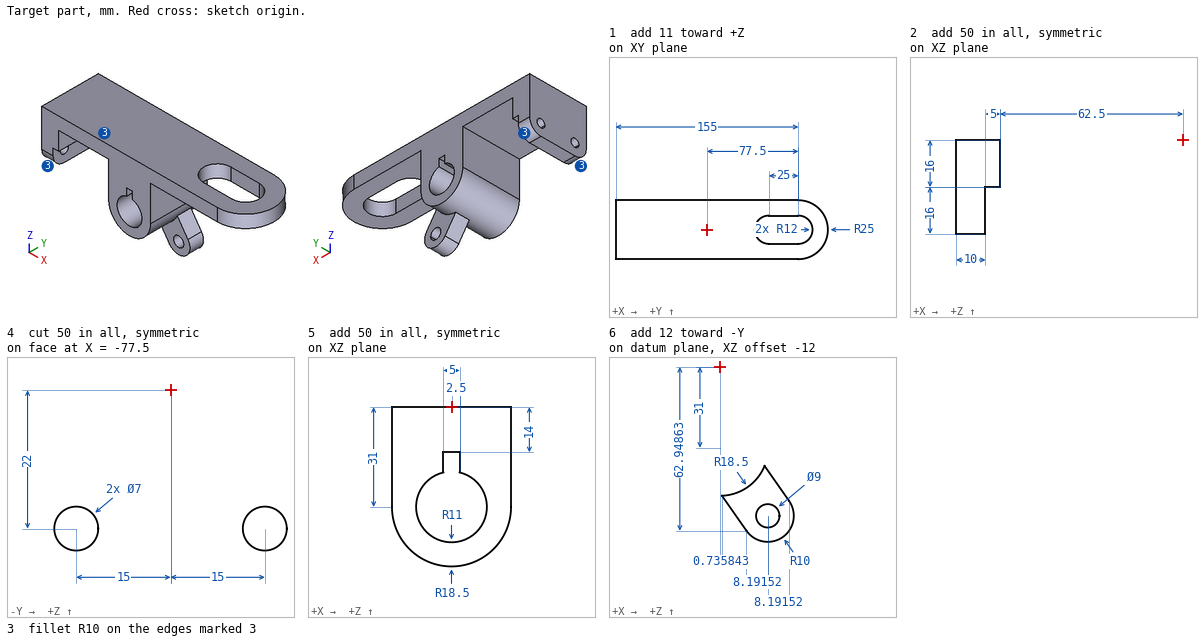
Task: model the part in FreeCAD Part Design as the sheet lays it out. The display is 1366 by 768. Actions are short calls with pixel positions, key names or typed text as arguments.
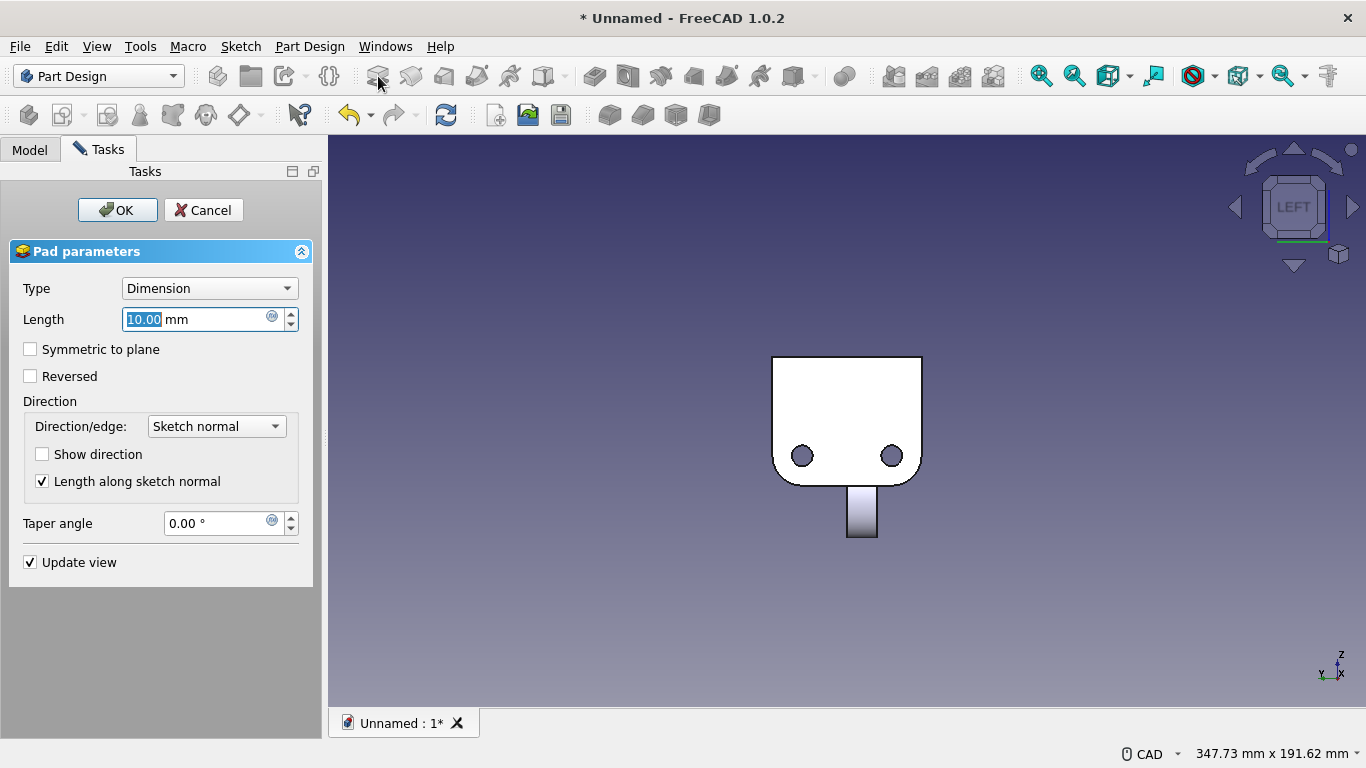
text(50)
key(Tab)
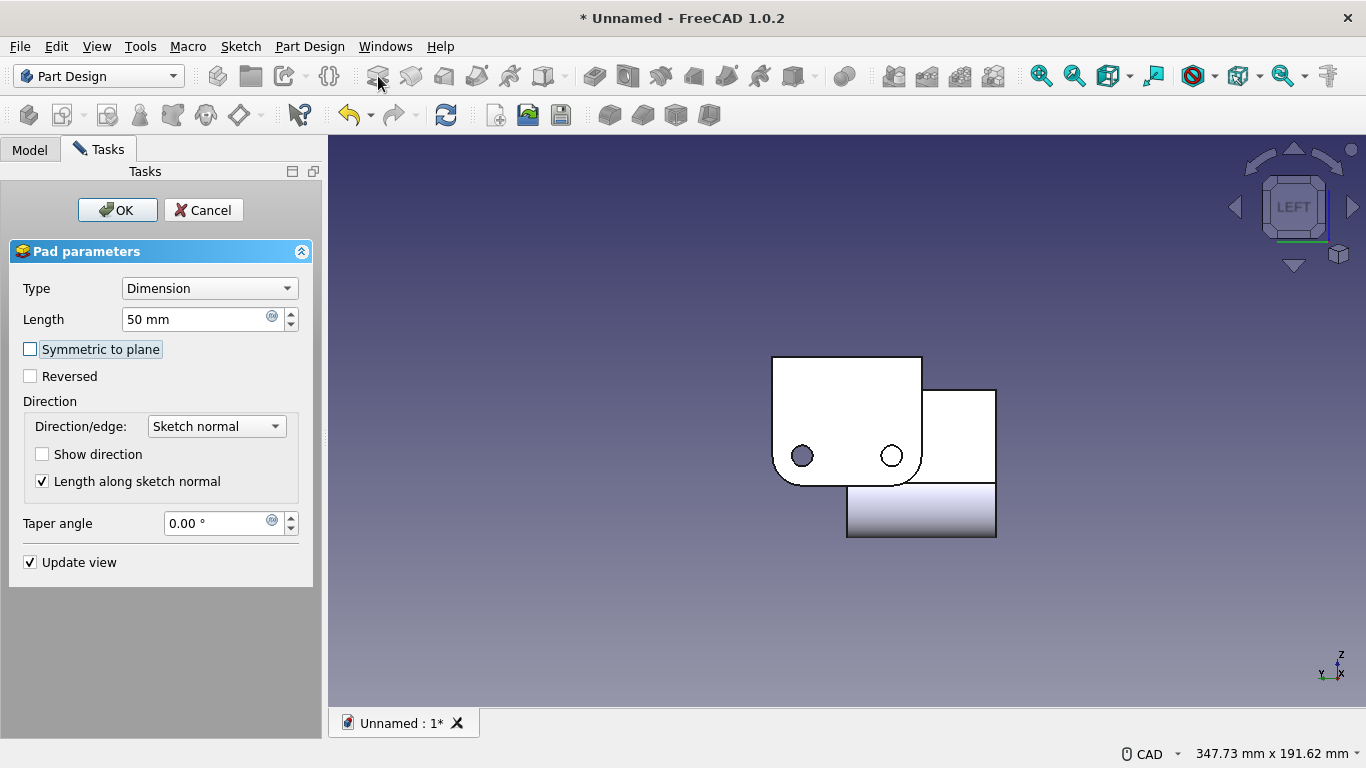
click(31, 349)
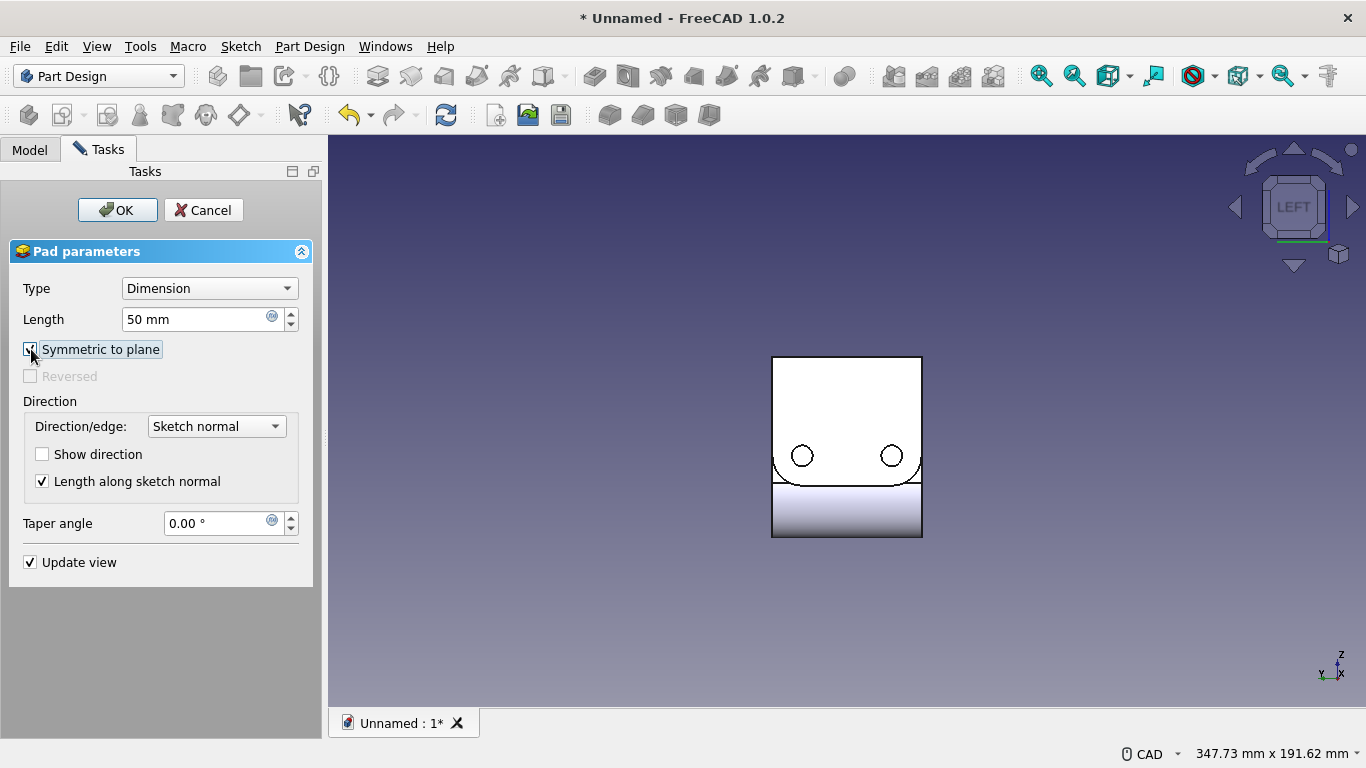
click(118, 210)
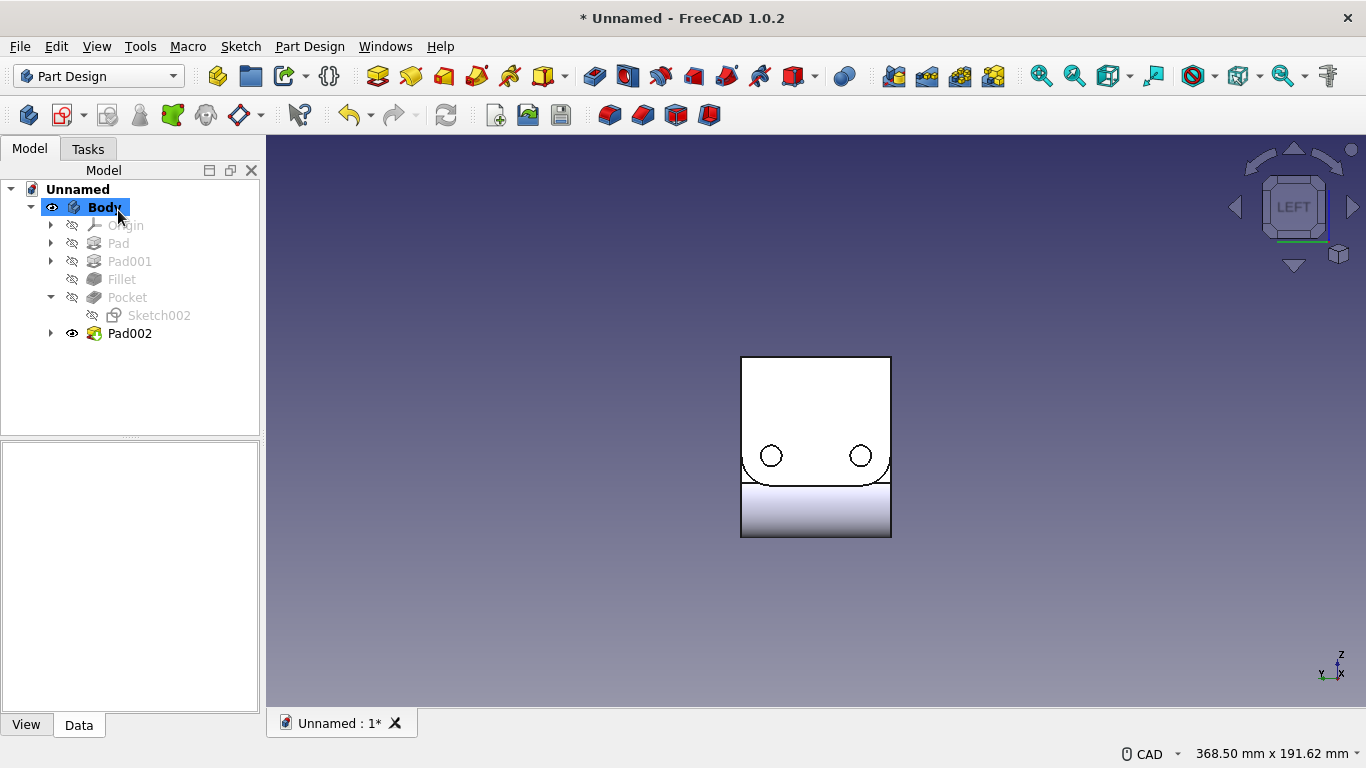
click(1042, 76)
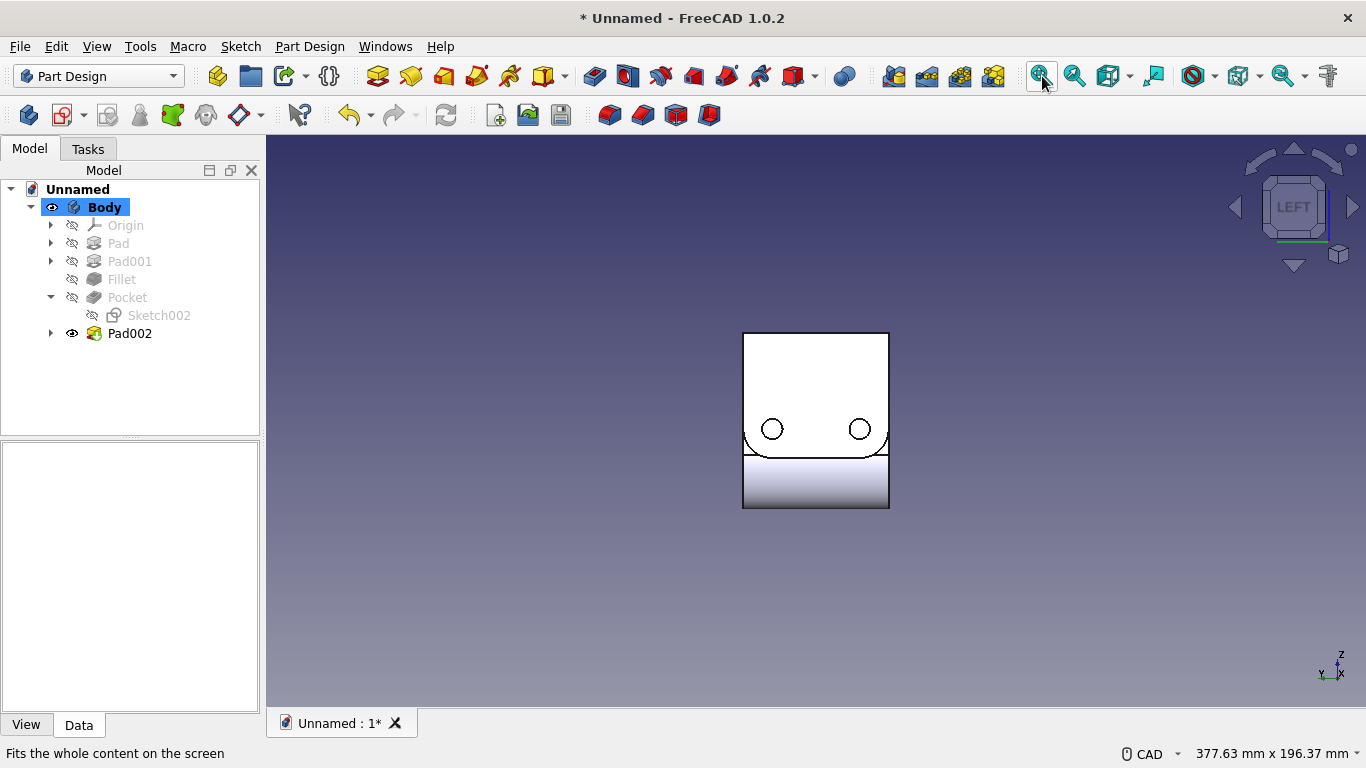
click(51, 225)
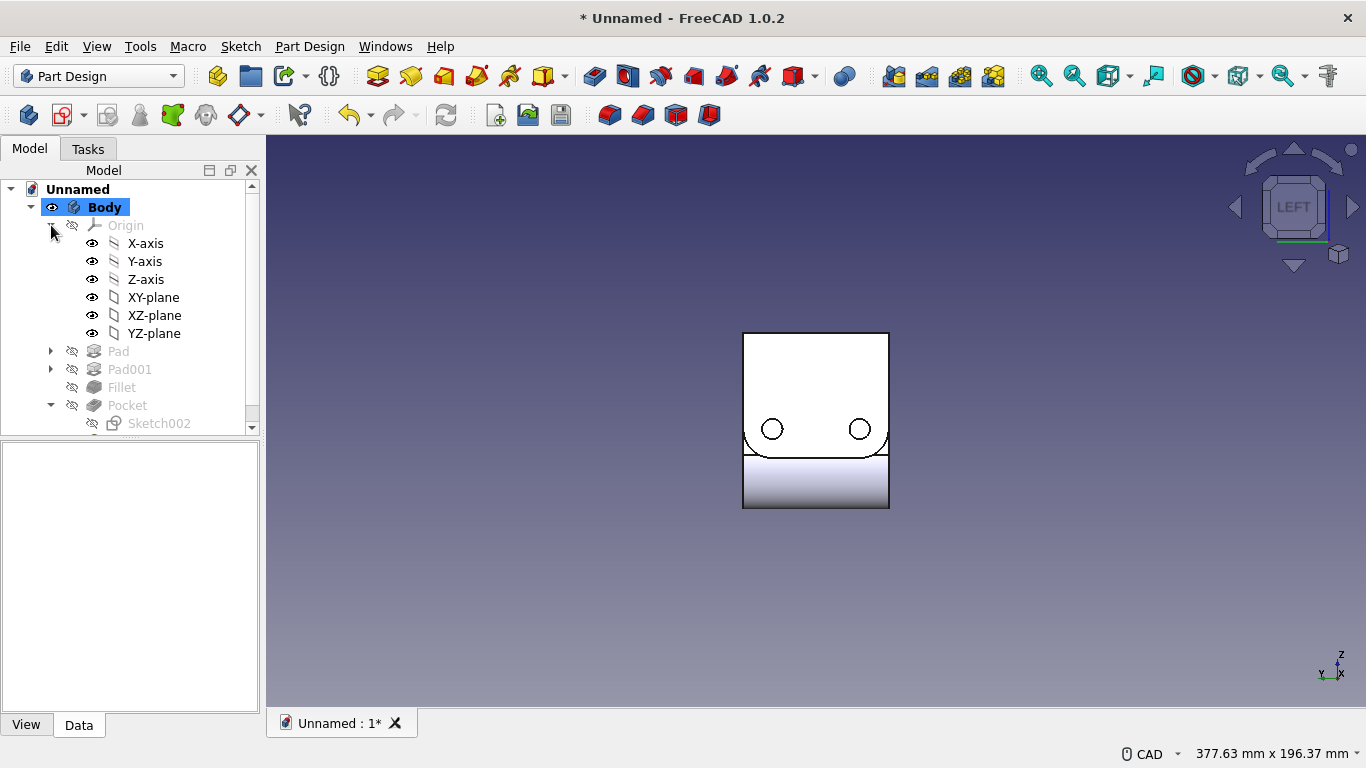
click(137, 315)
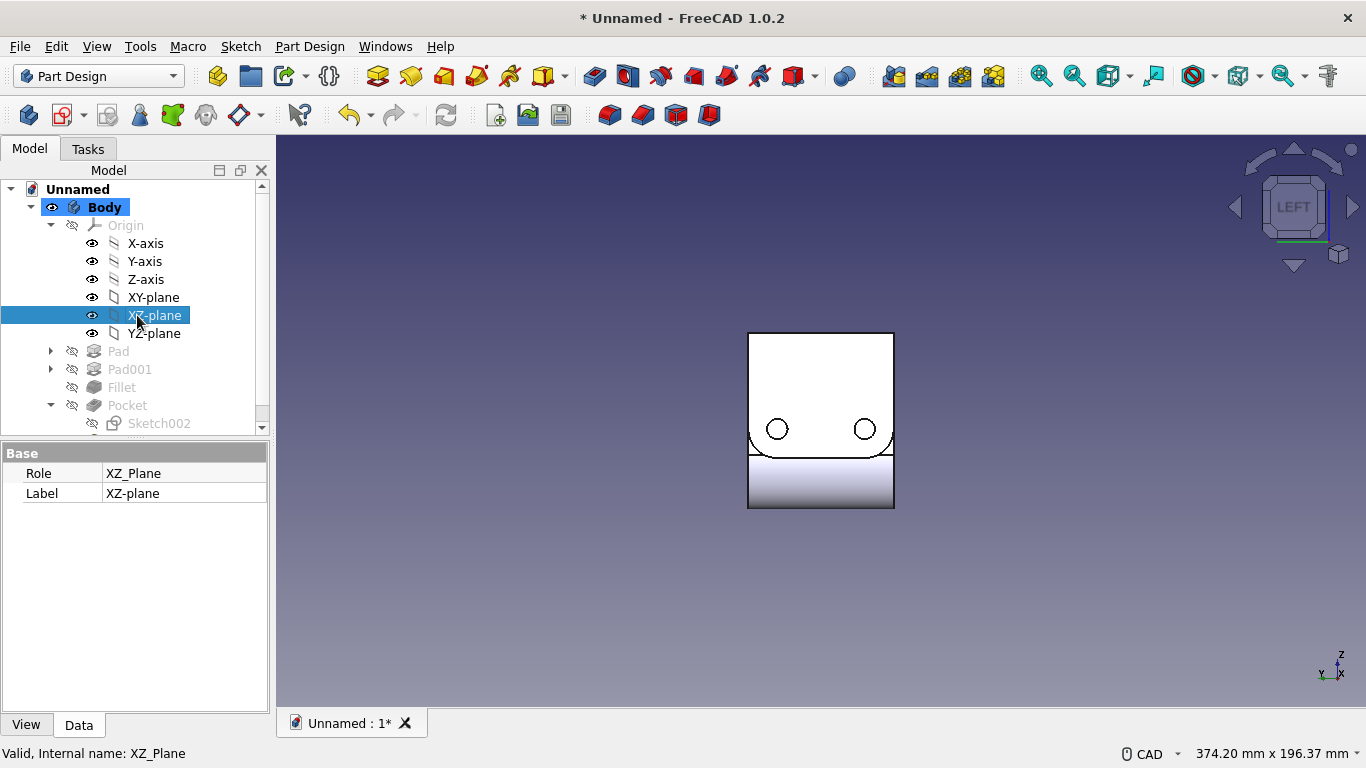
click(238, 116)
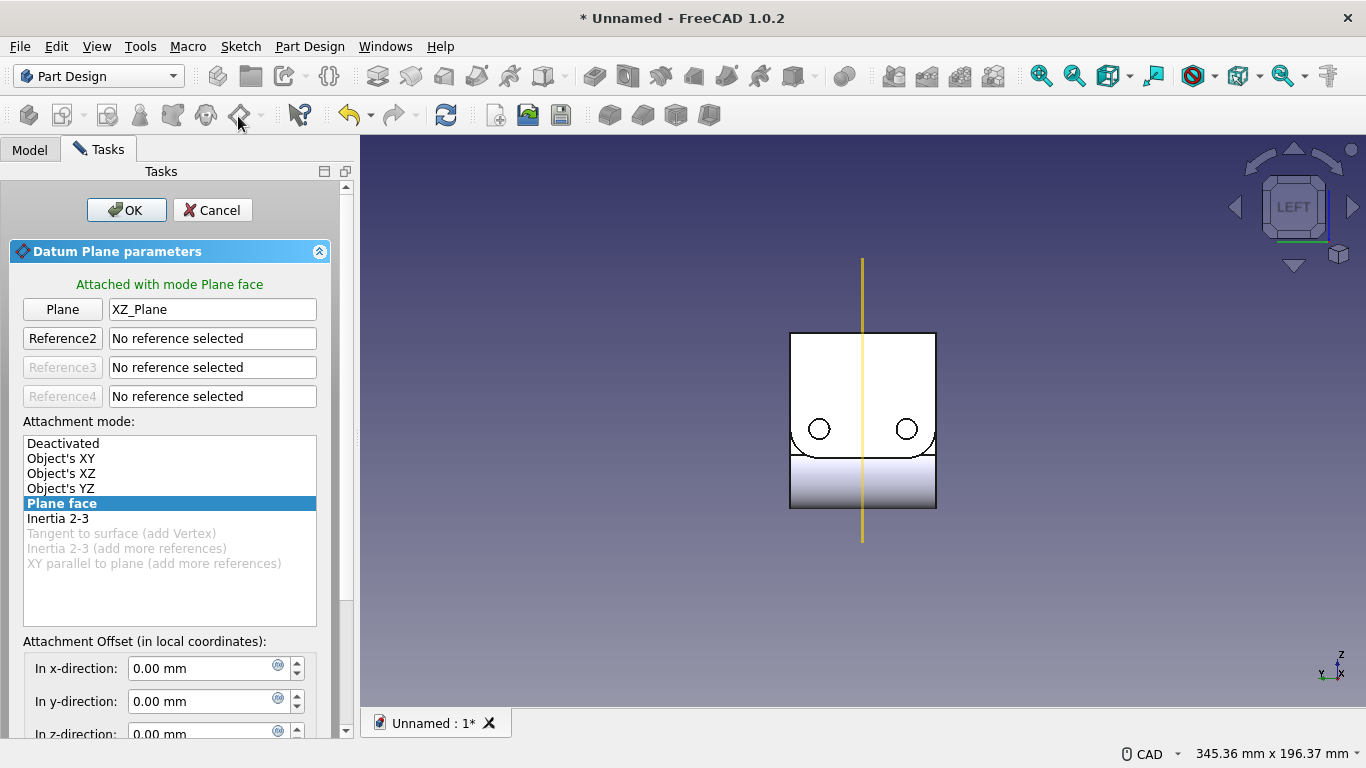
scroll(346, 460, down, 2)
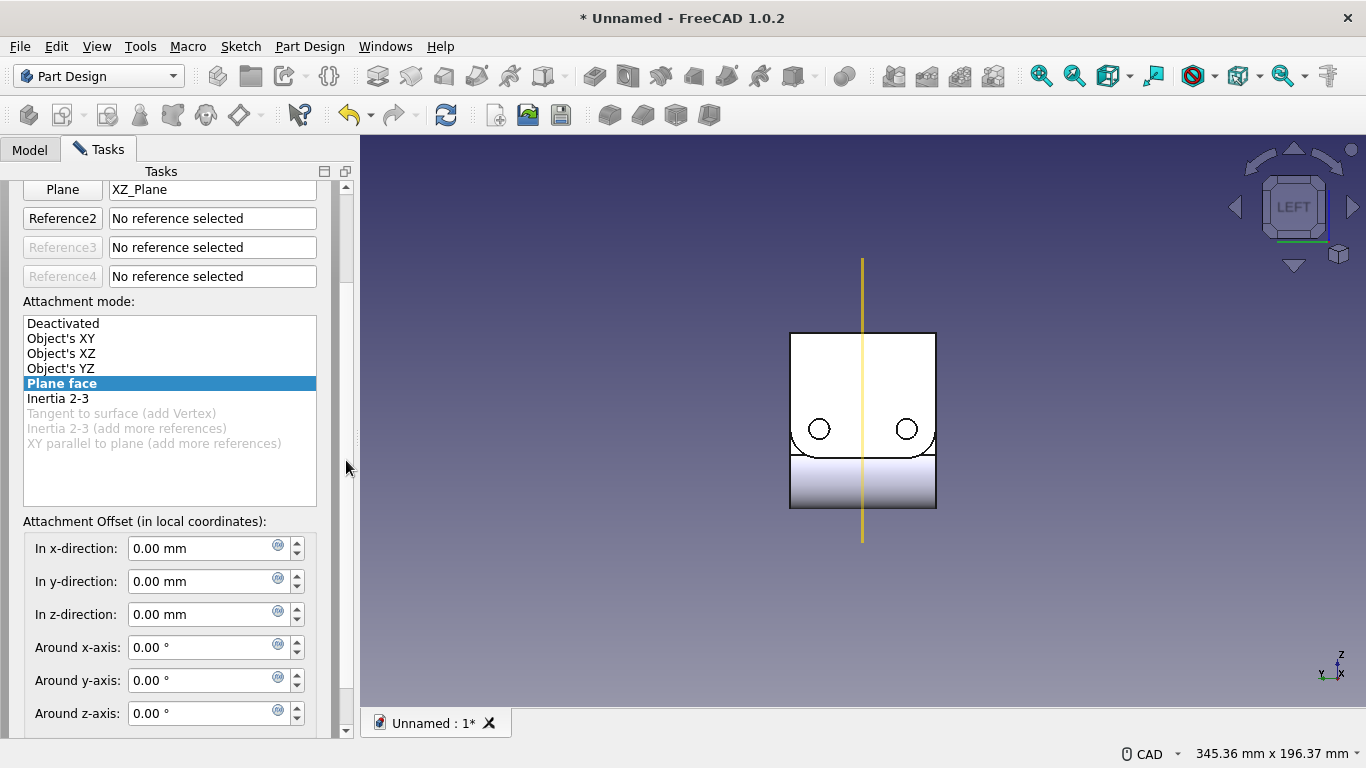
triple_click(210, 614)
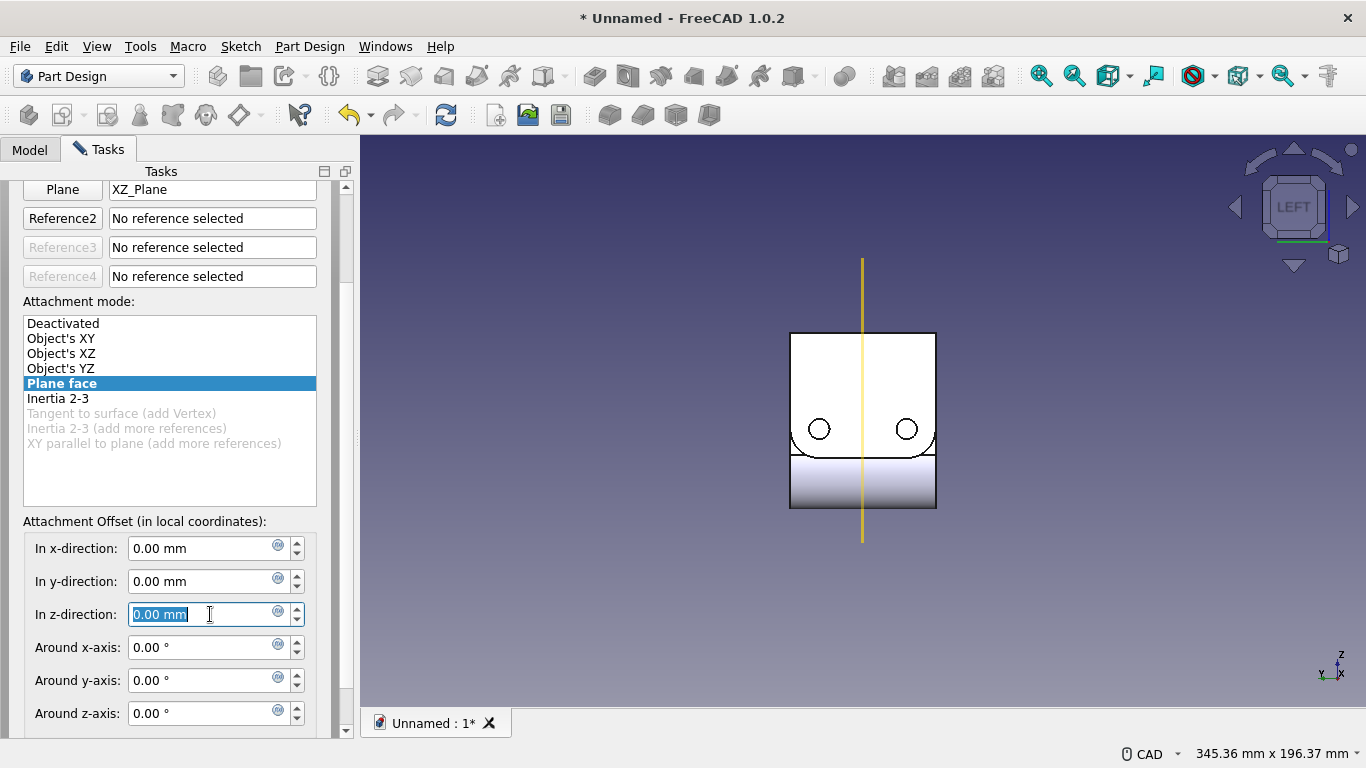
text(-12)
key(Tab)